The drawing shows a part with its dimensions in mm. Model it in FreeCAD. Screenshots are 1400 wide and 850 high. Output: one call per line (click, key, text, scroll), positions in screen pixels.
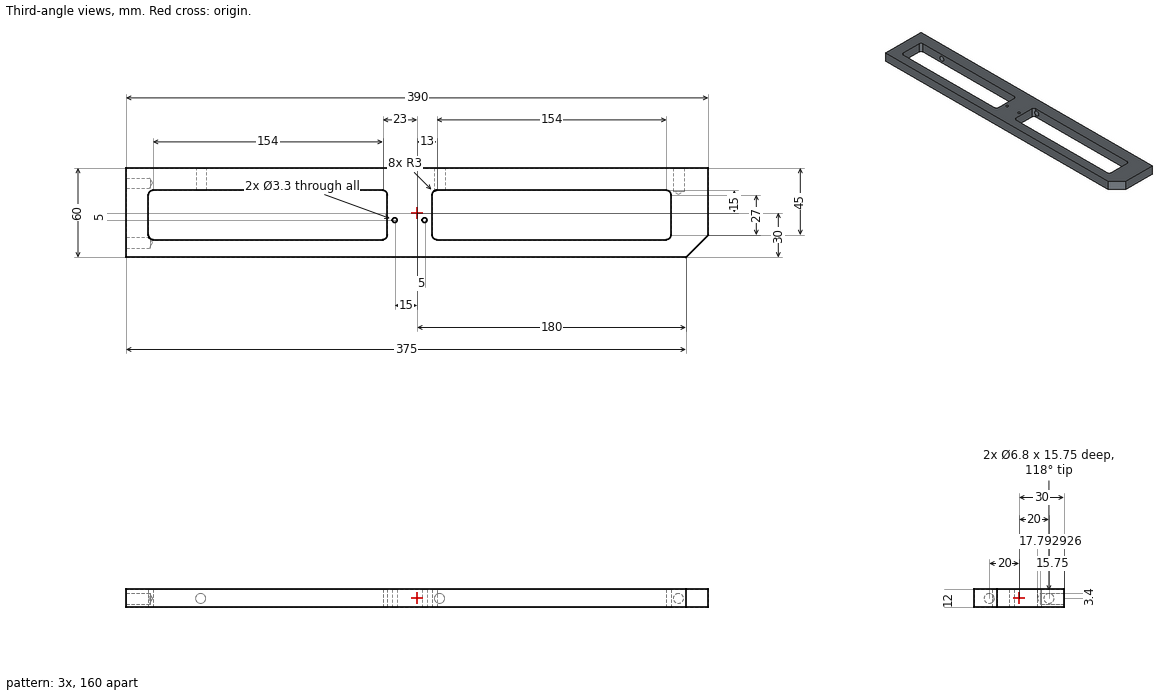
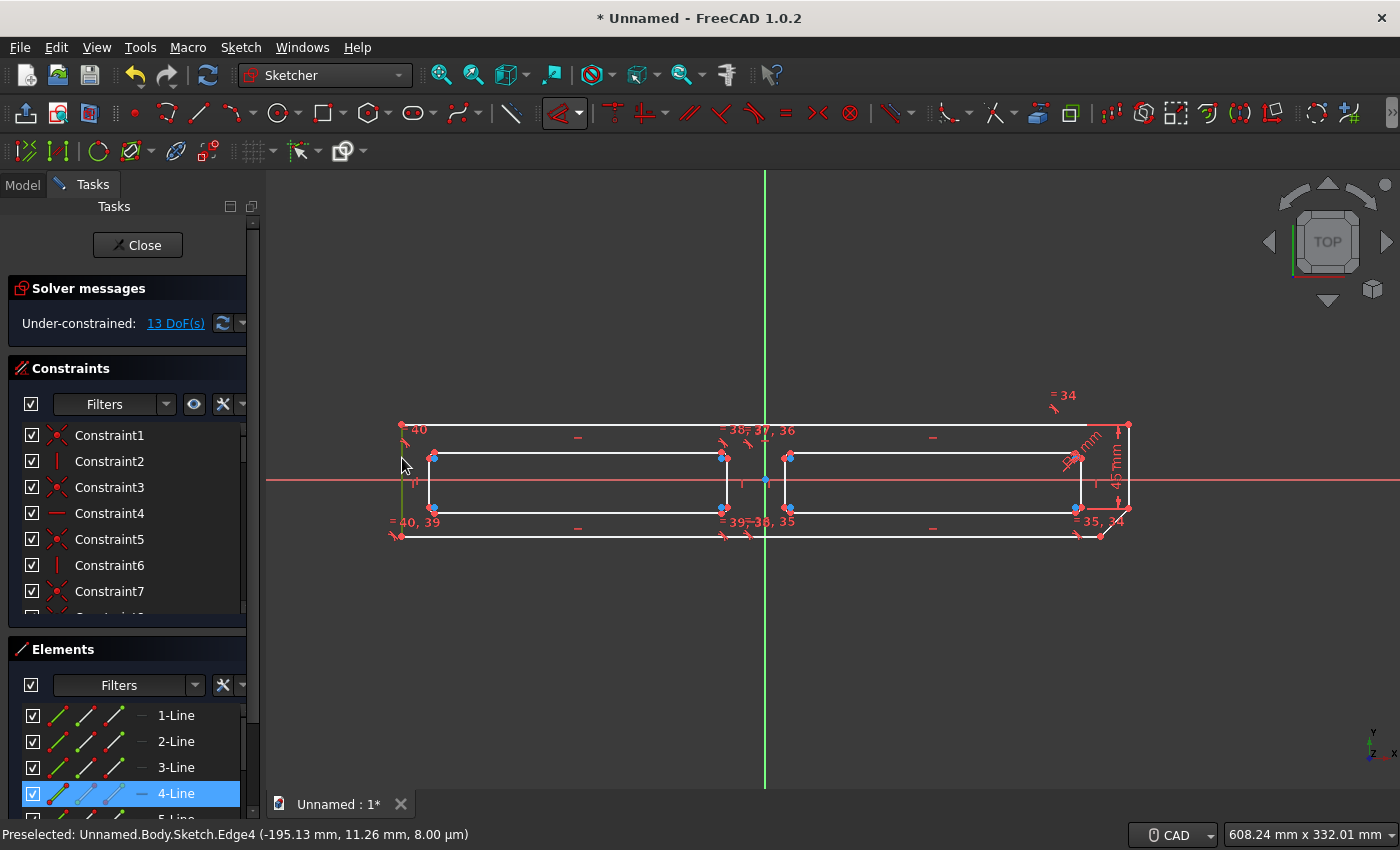
key(i)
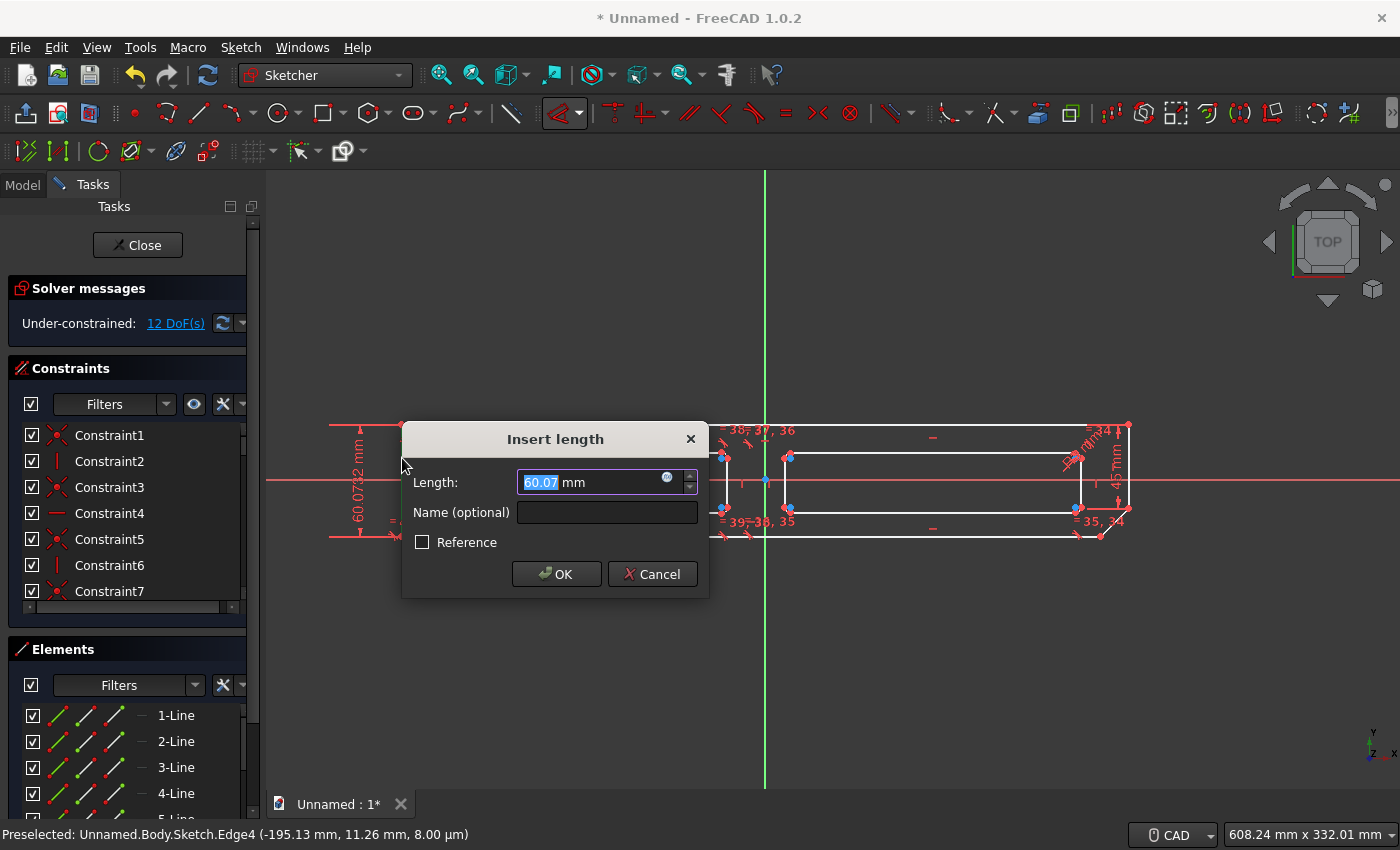
text(60)
key(Return)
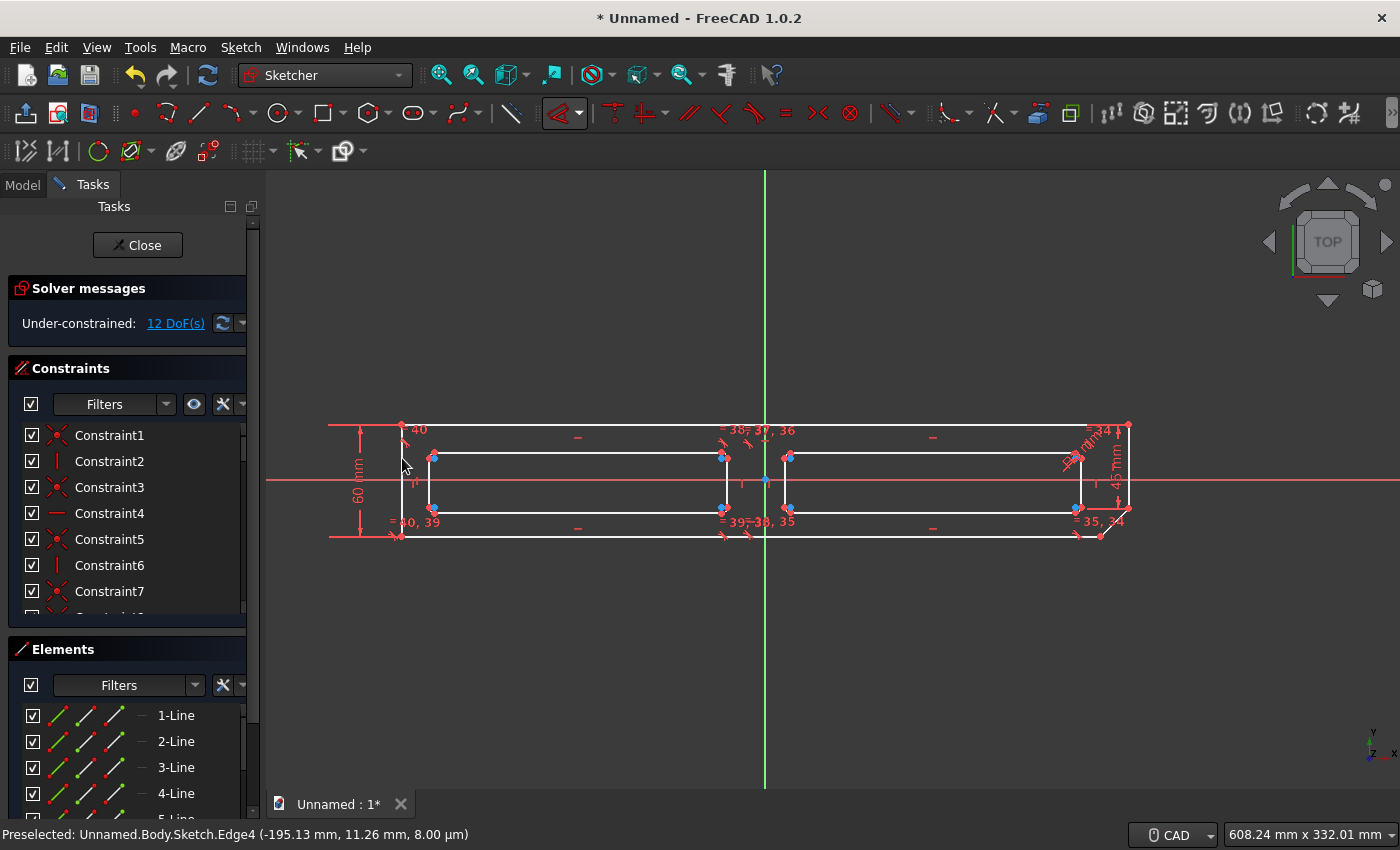
click(1081, 493)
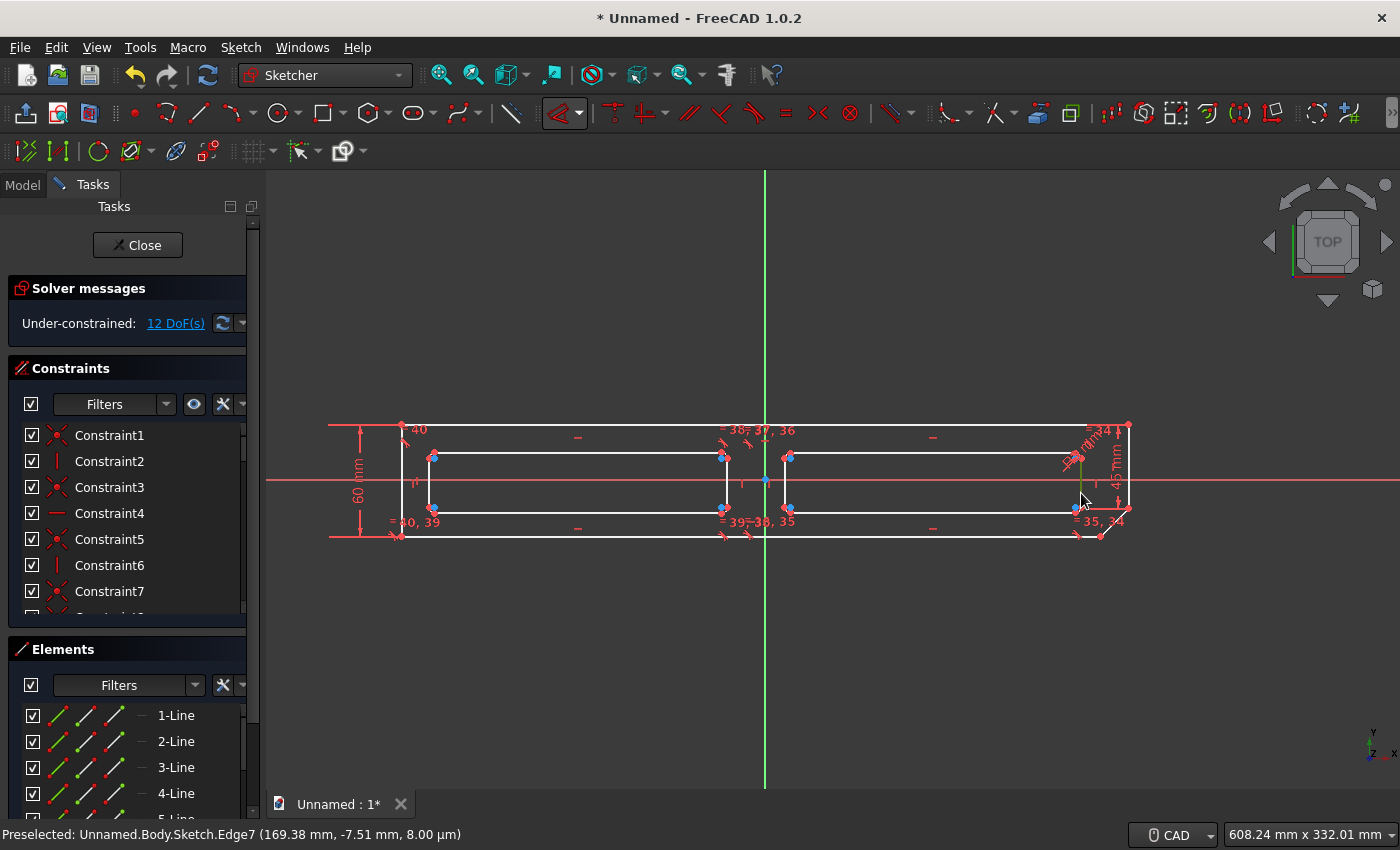
click(582, 114)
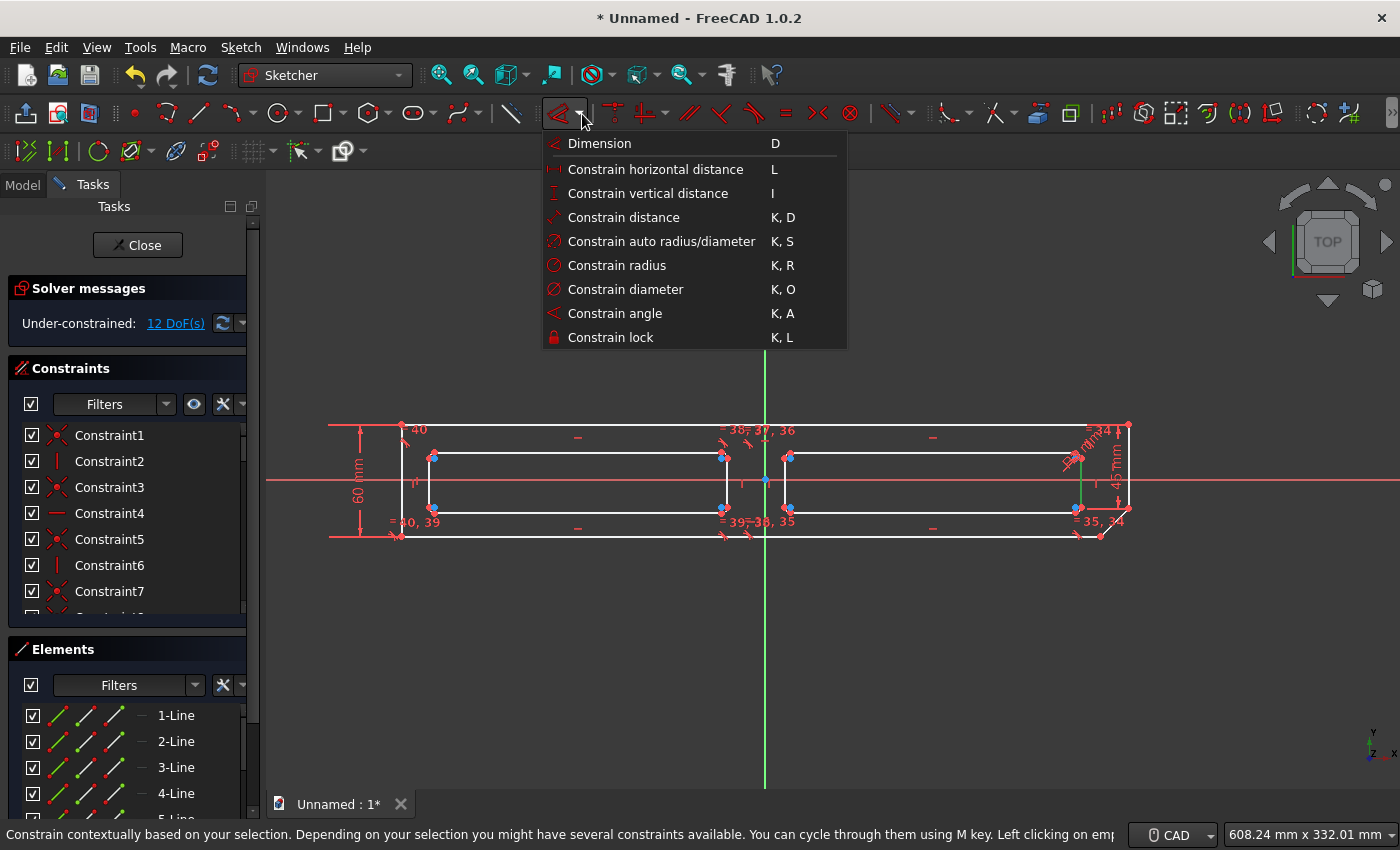
click(695, 193)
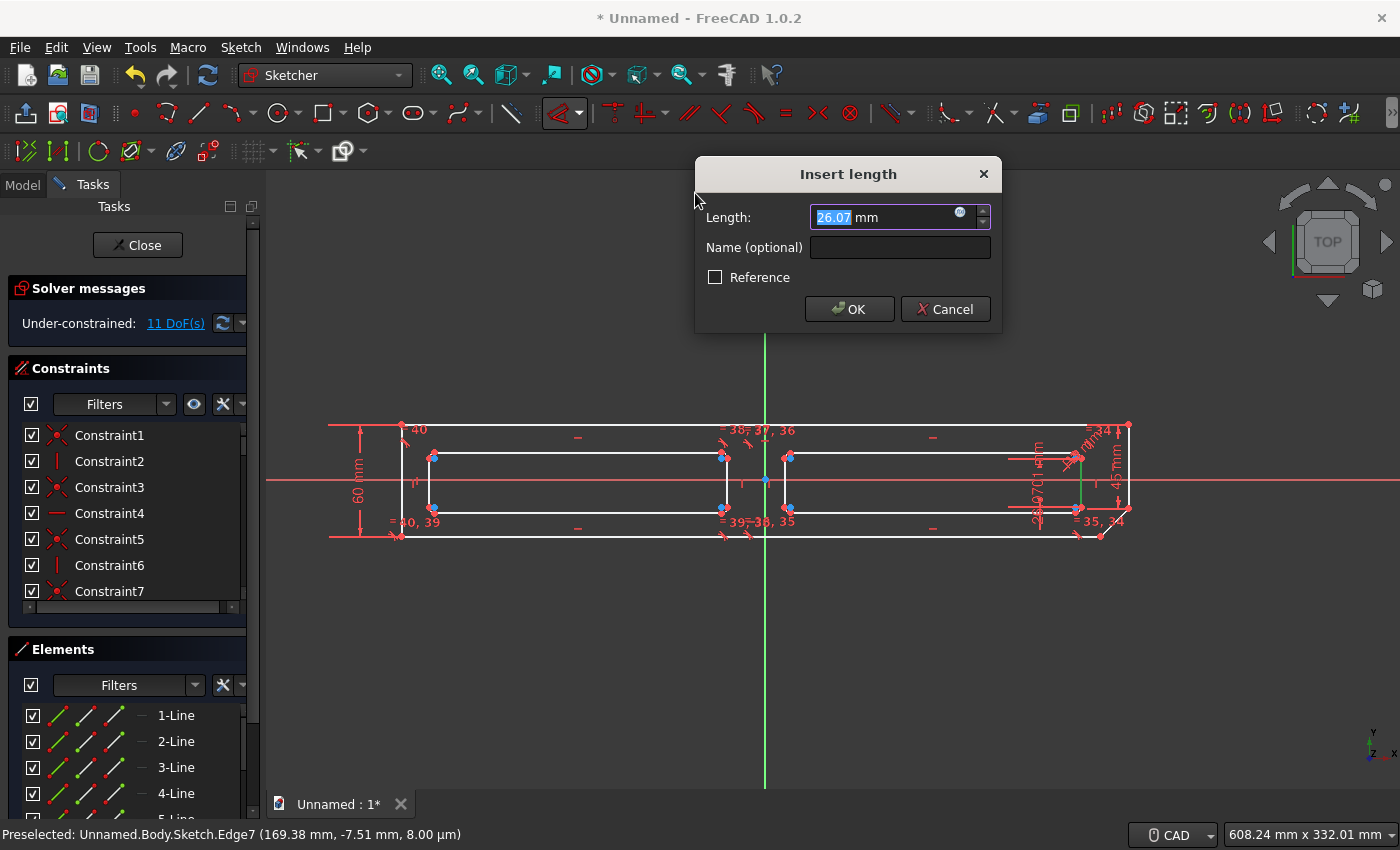
text(27)
key(Return)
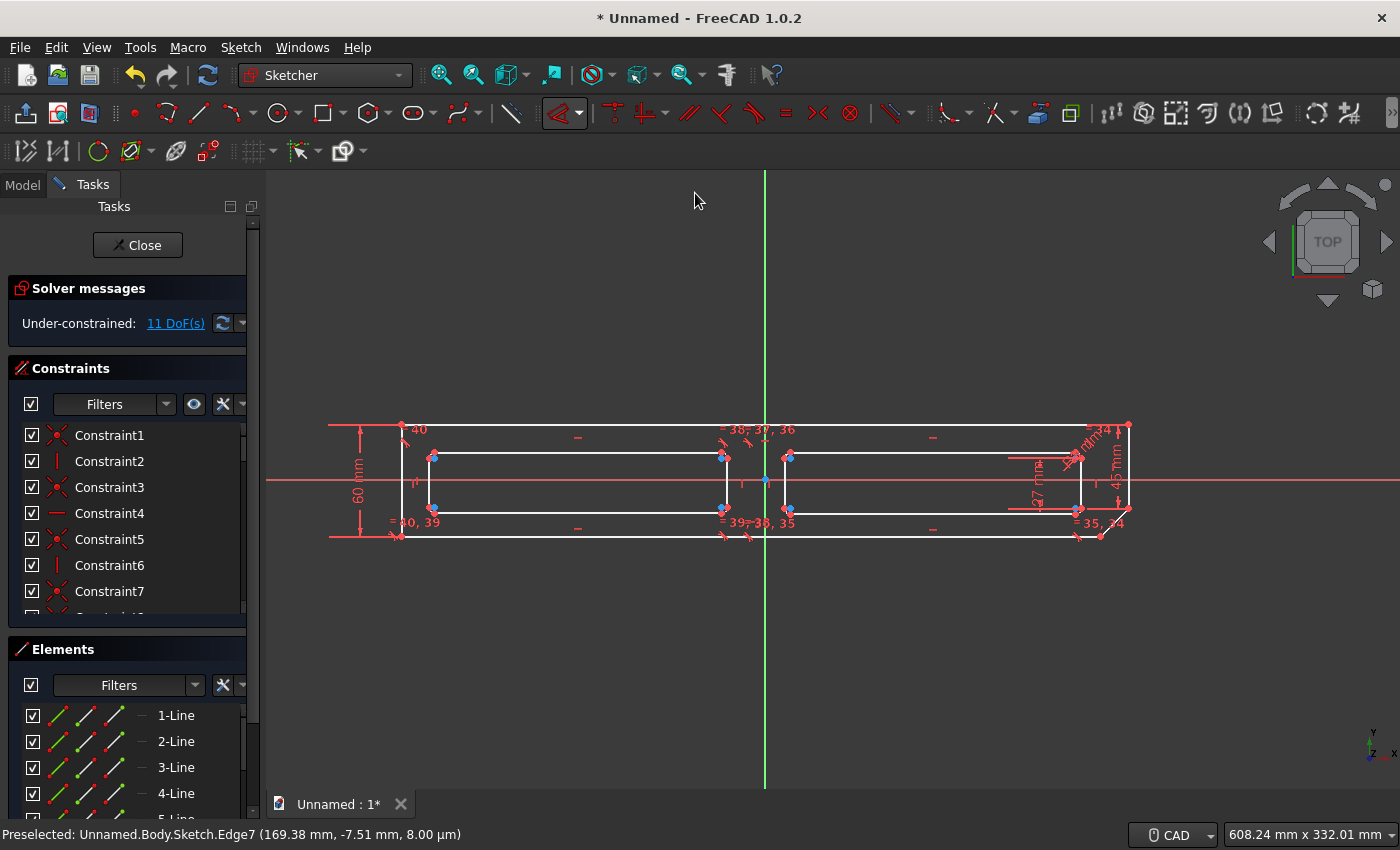
click(727, 493)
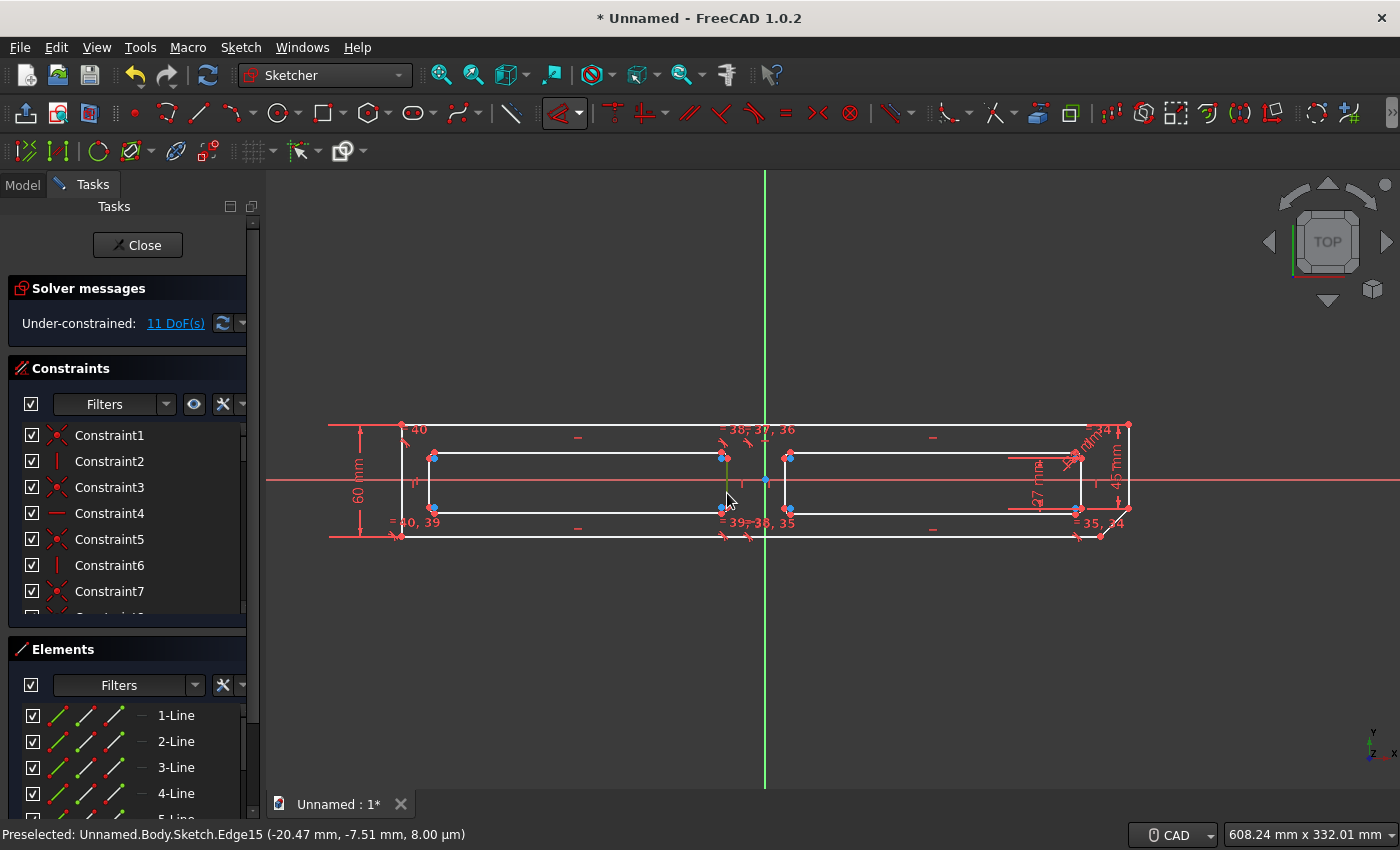
key(i)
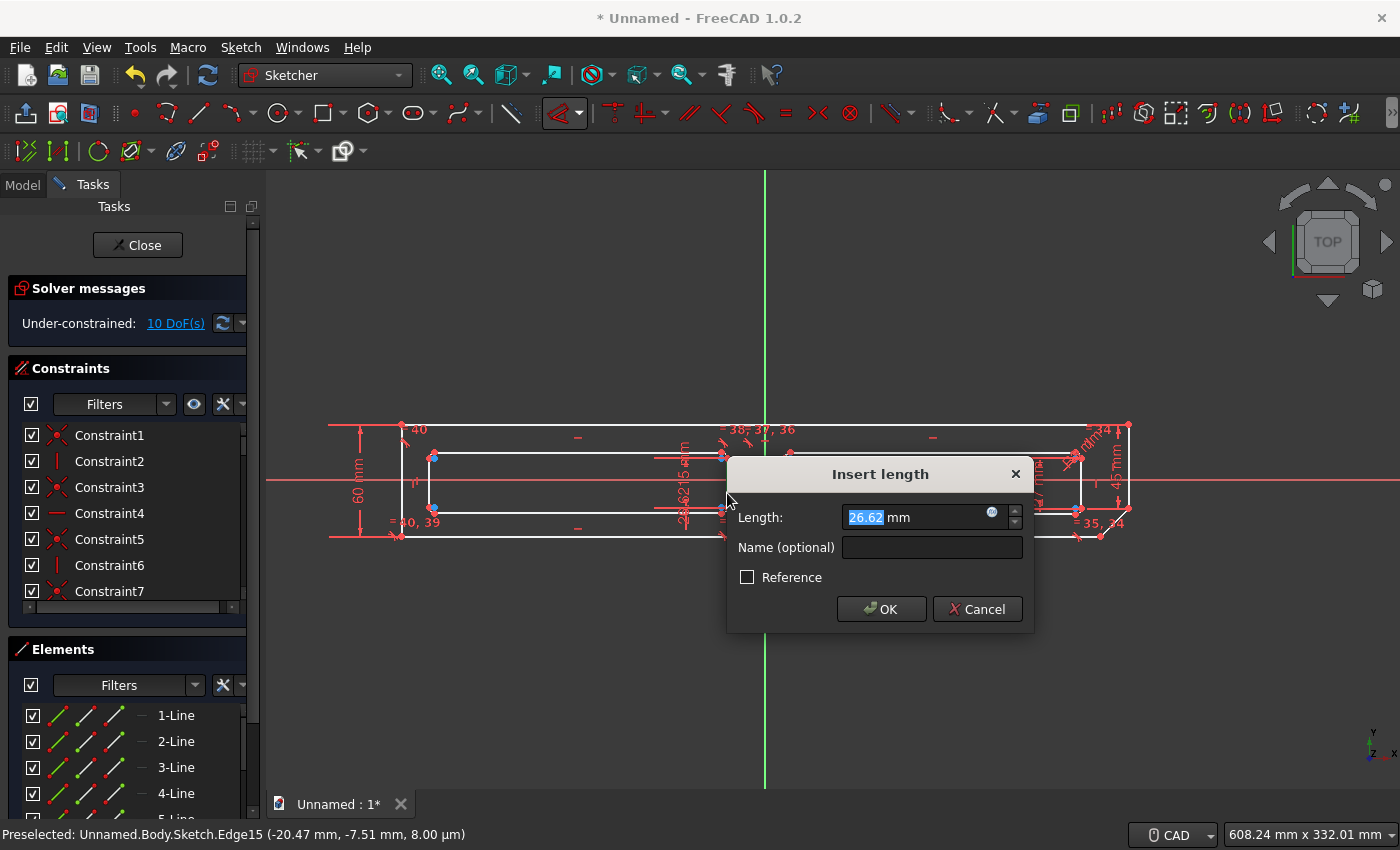
text(27)
key(Return)